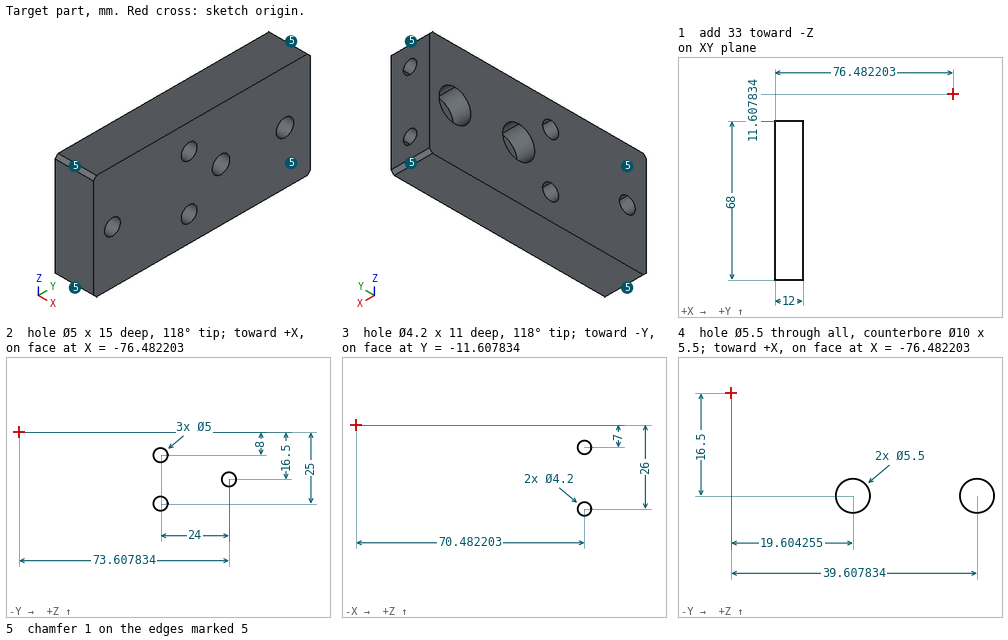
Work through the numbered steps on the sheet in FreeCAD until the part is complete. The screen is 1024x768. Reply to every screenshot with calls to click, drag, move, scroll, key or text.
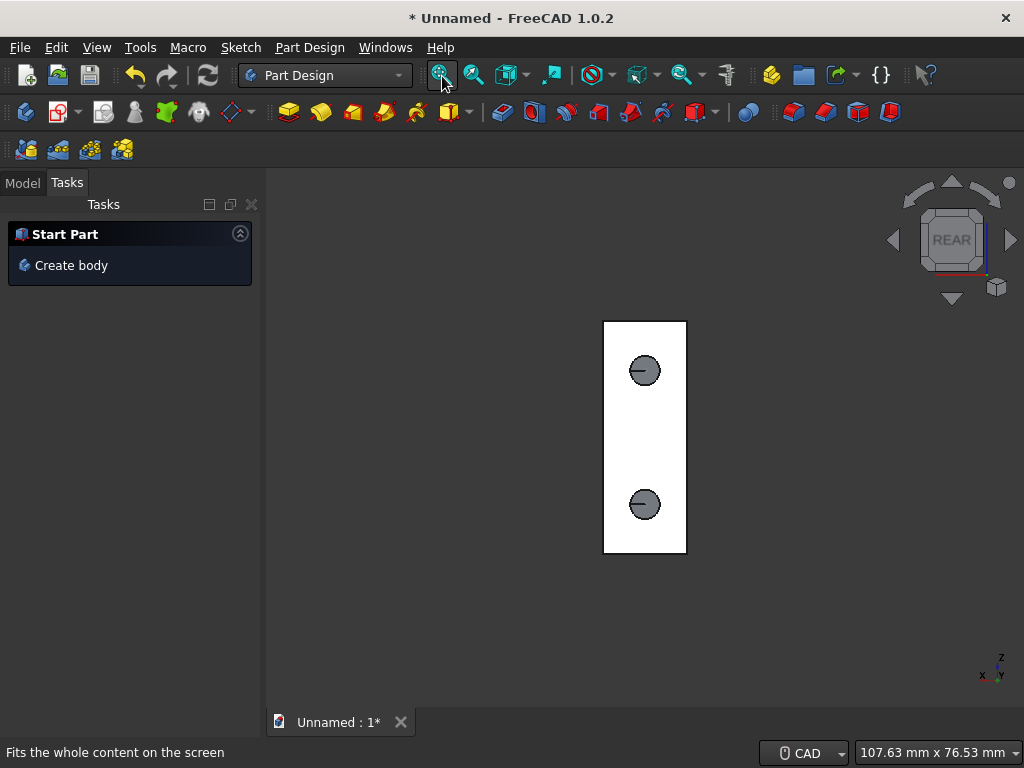
key(6)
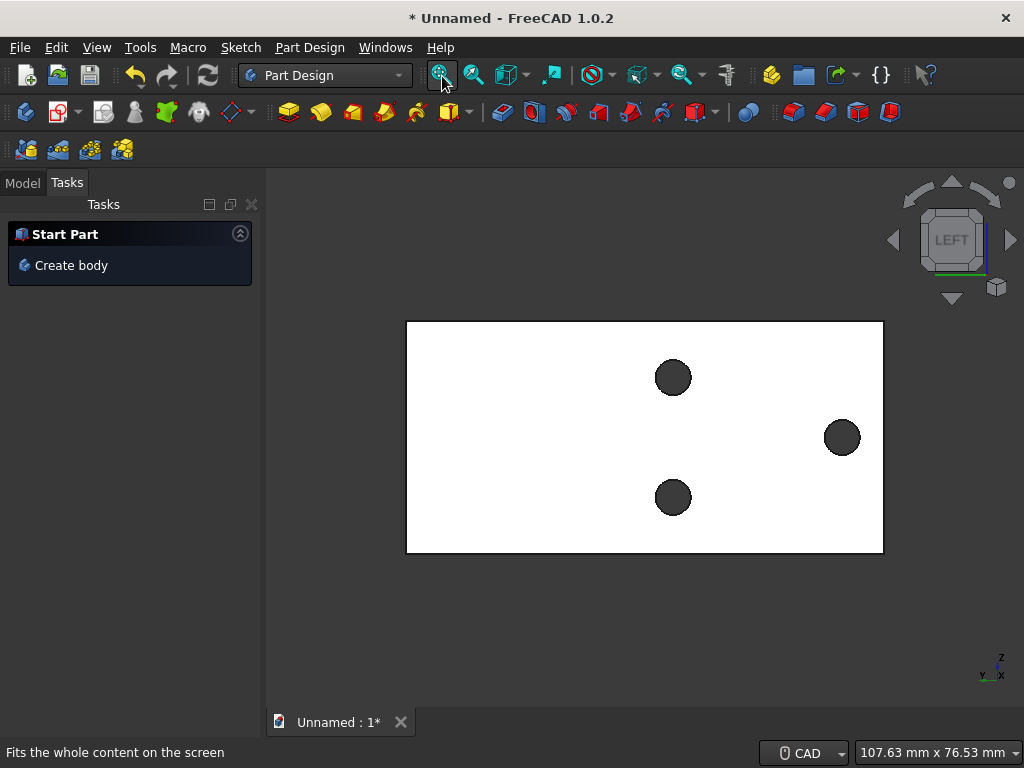
click(508, 436)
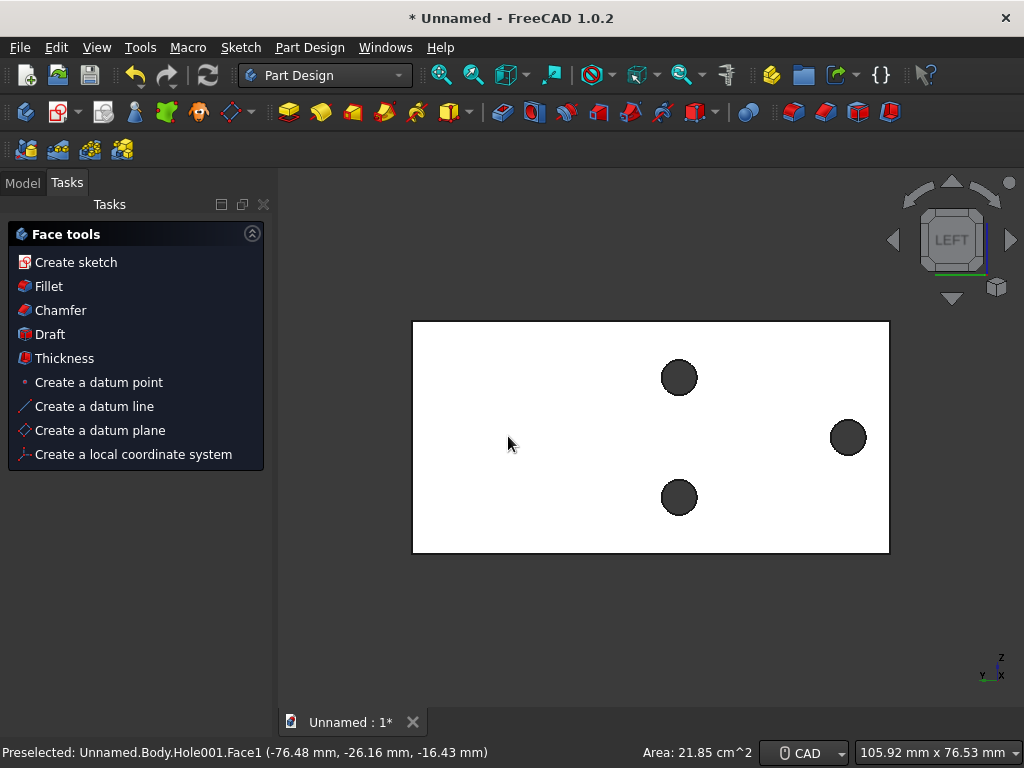
click(58, 112)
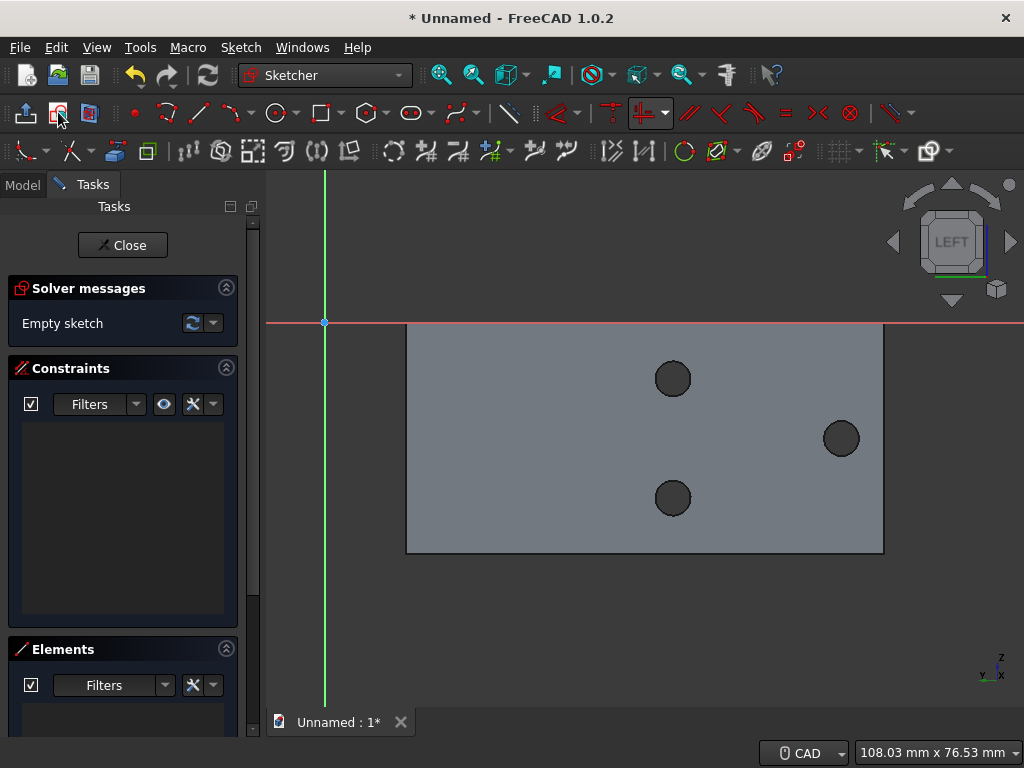
key(g)
key(c)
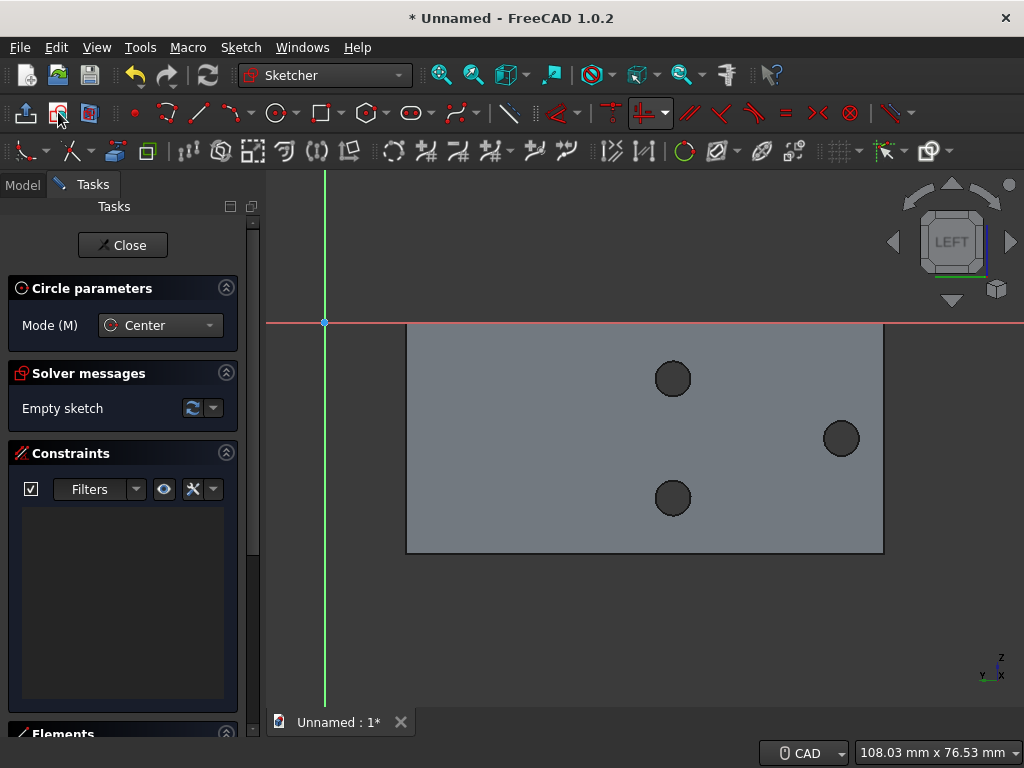
click(463, 438)
click(476, 425)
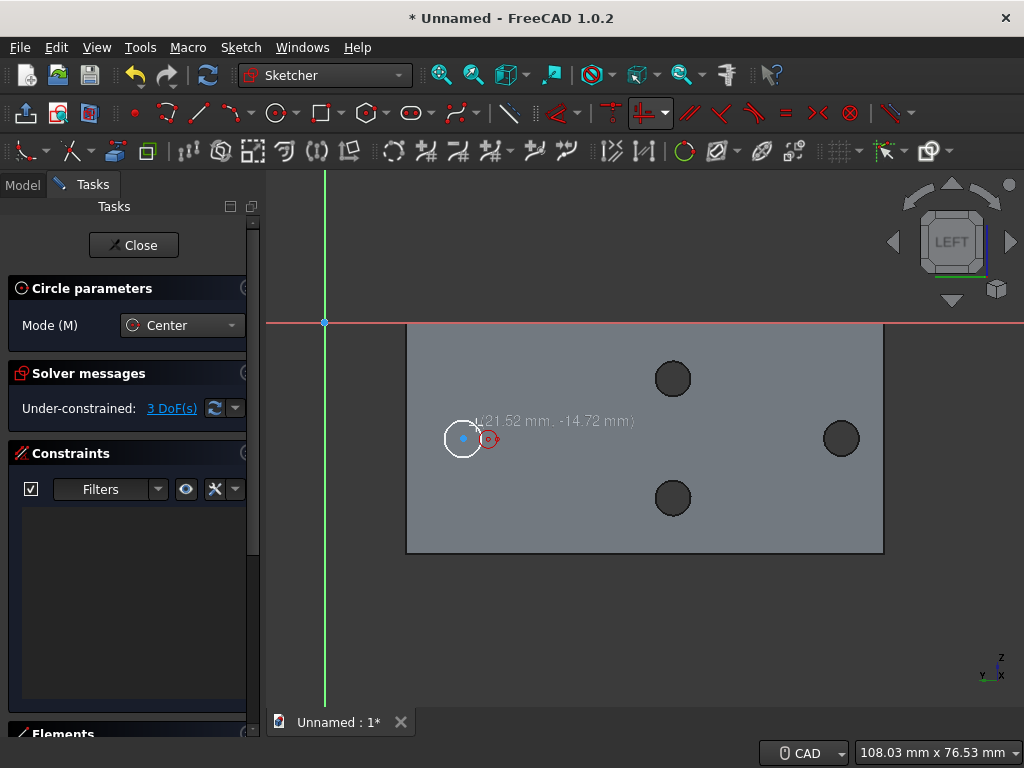
click(603, 438)
click(617, 425)
key(Escape)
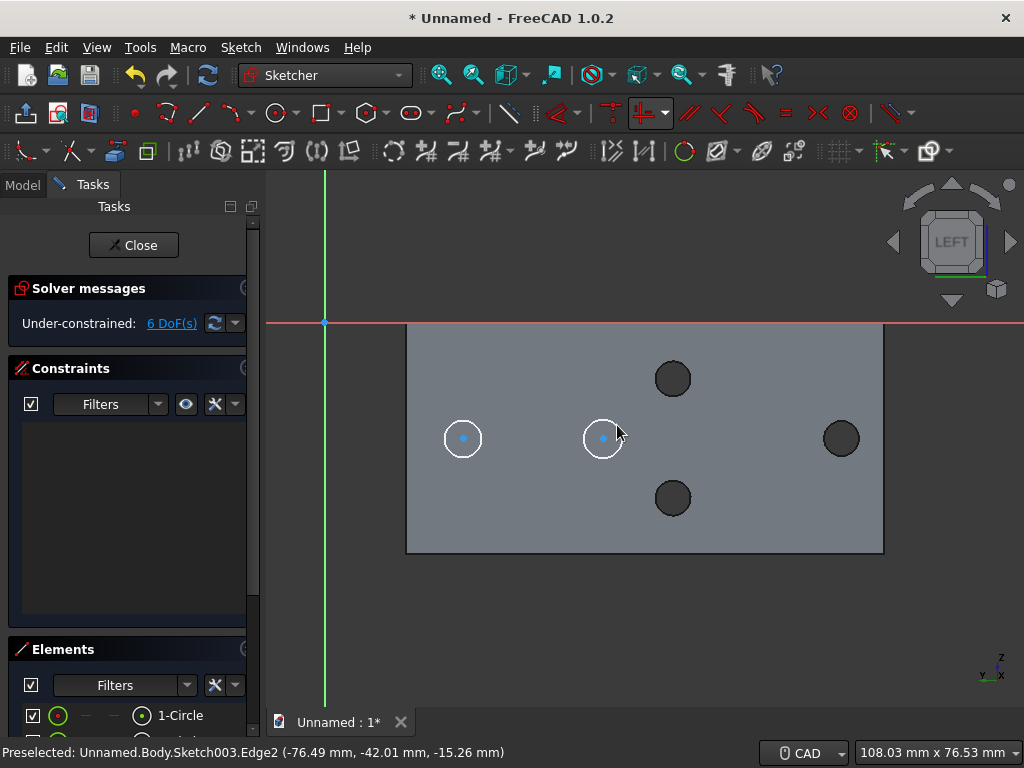
click(476, 426)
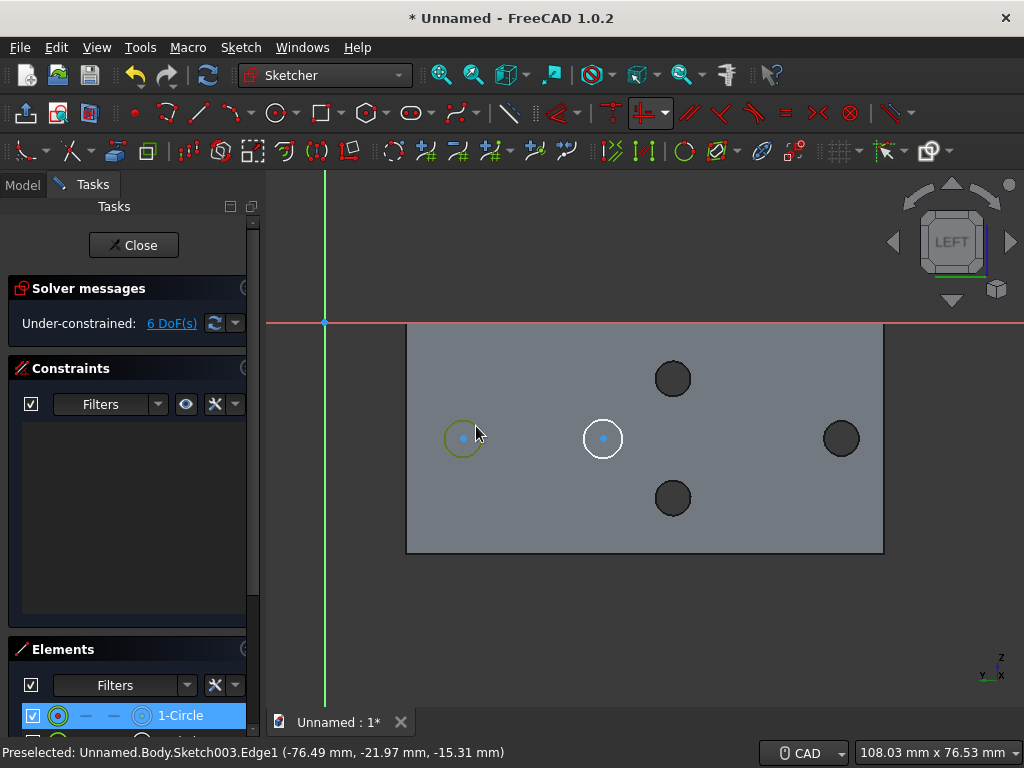
click(616, 425)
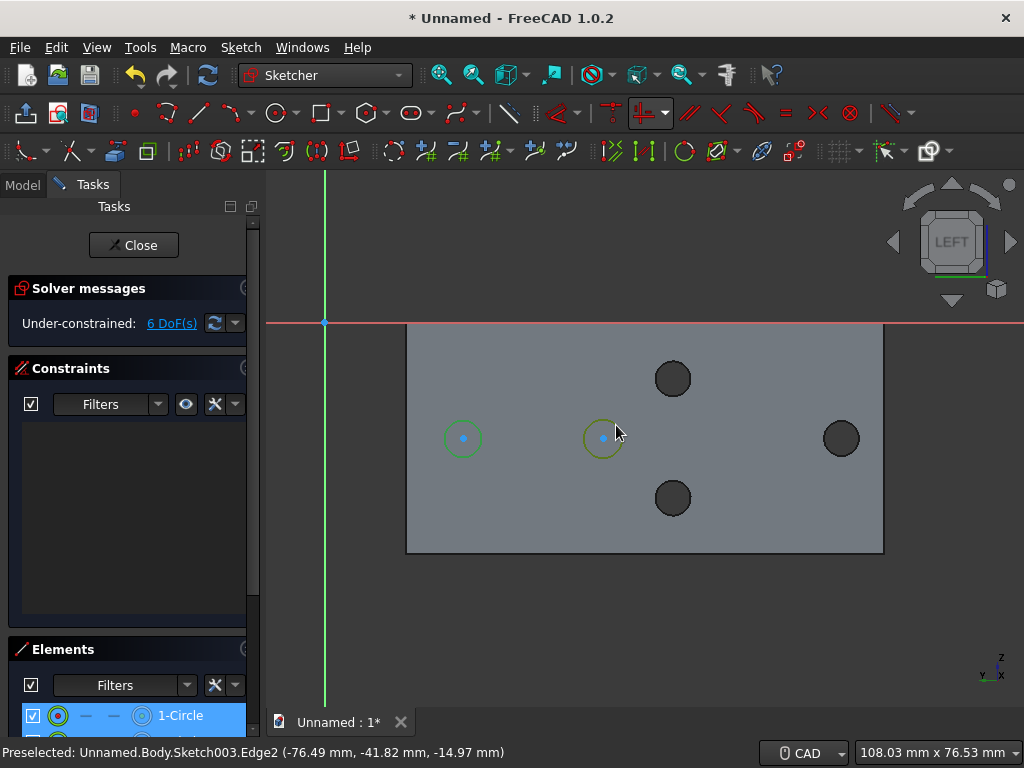
key(e)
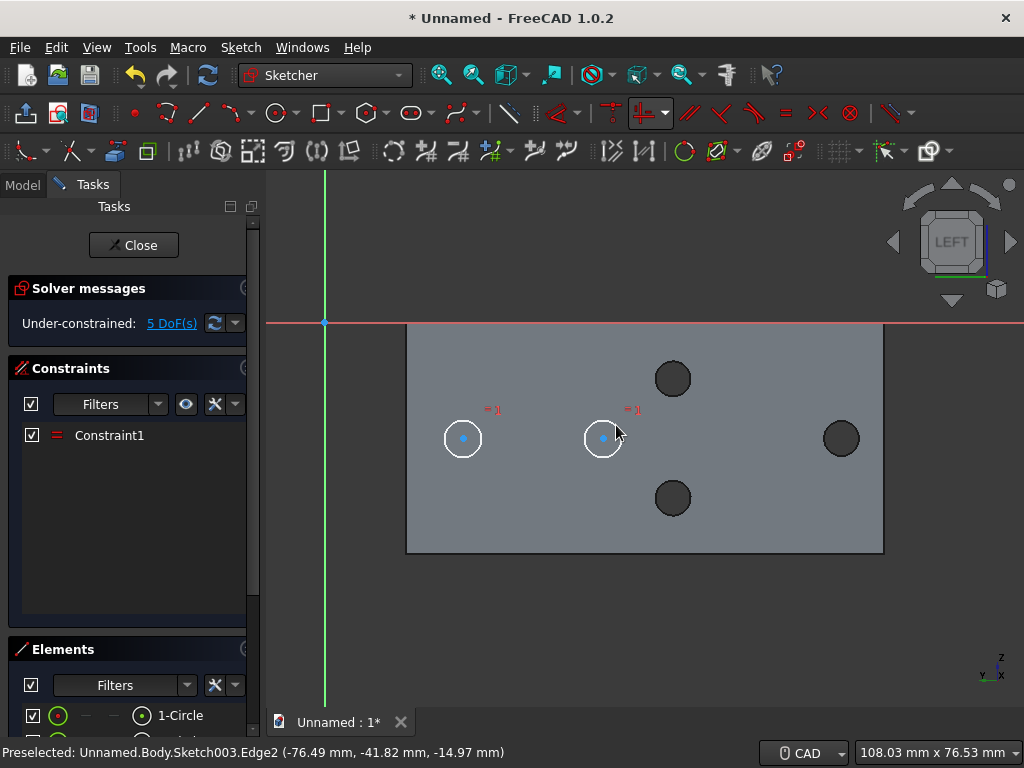
click(463, 439)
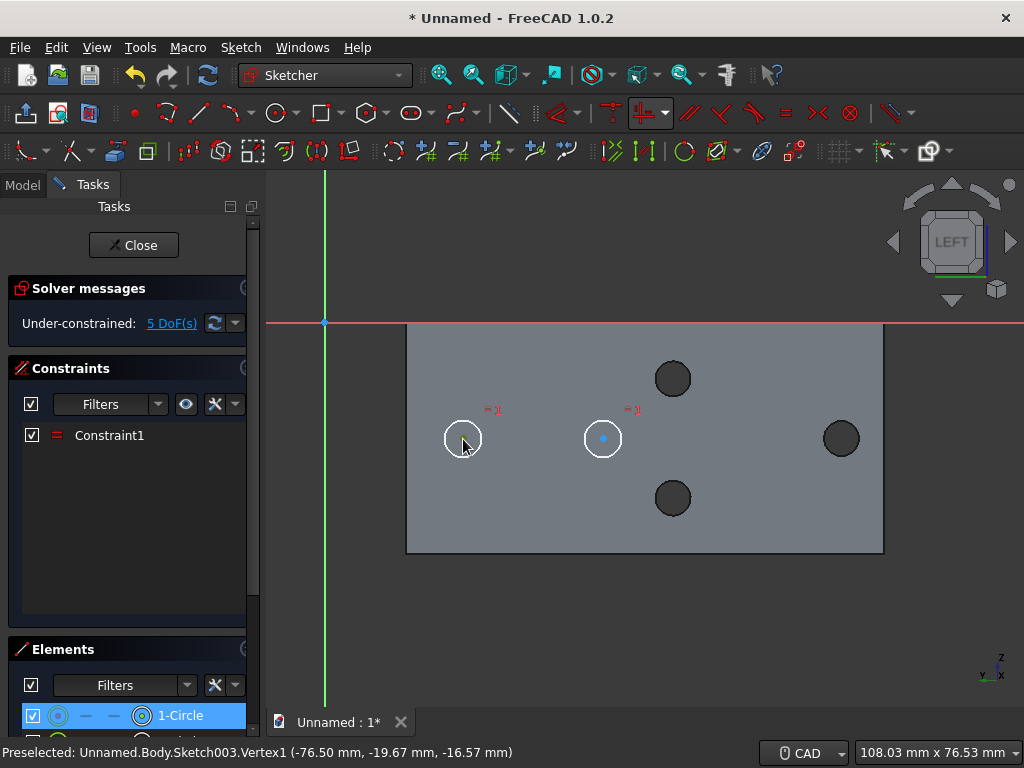
click(603, 439)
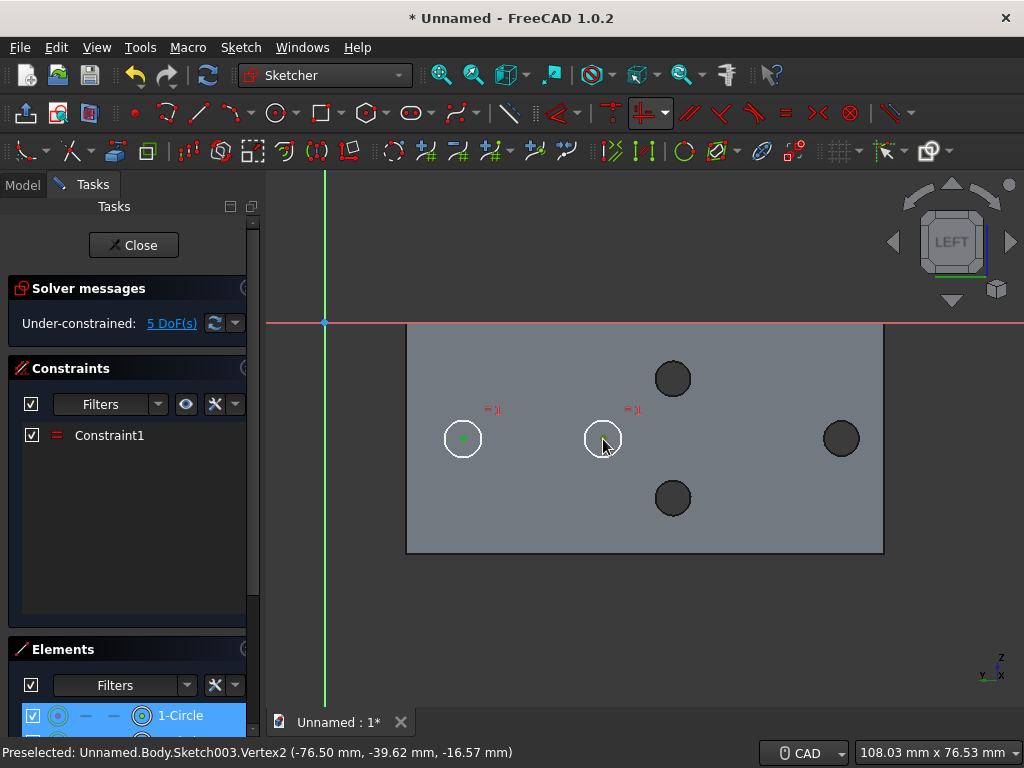
key(h)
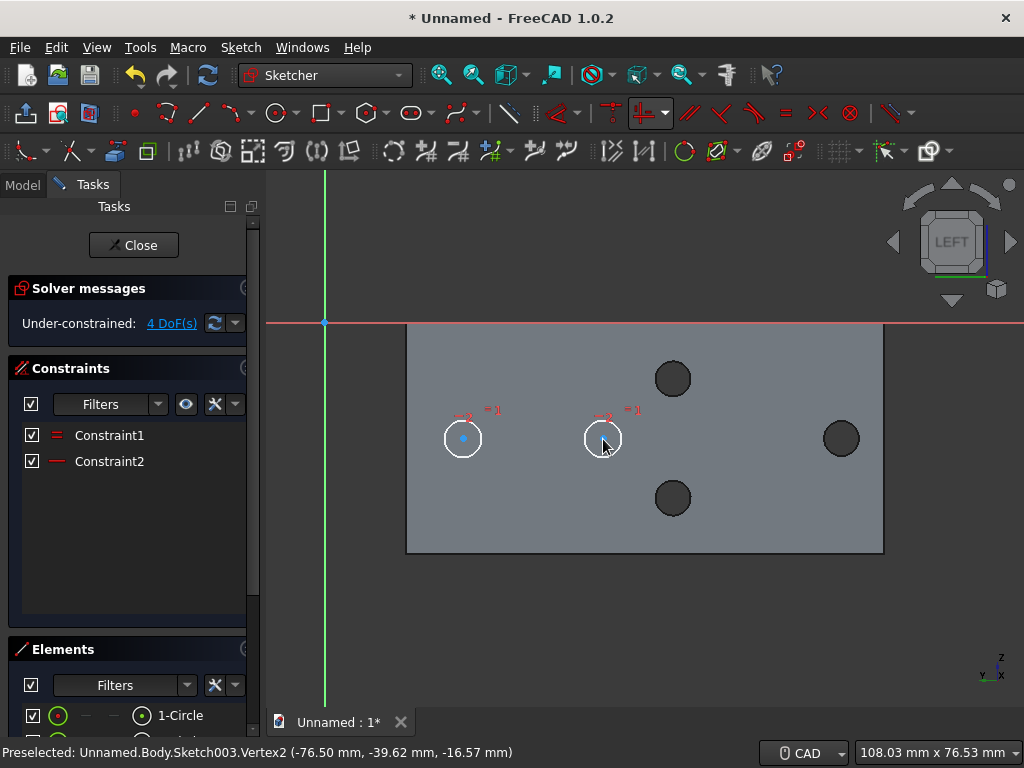
key(d)